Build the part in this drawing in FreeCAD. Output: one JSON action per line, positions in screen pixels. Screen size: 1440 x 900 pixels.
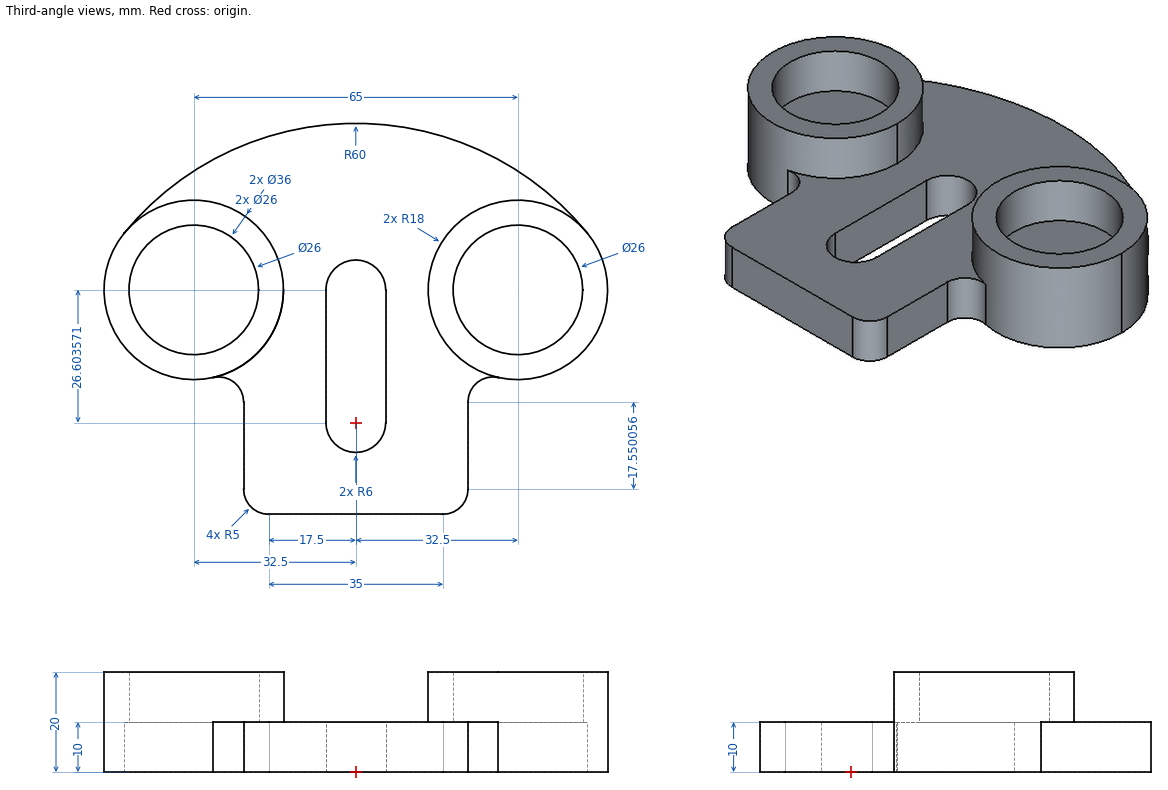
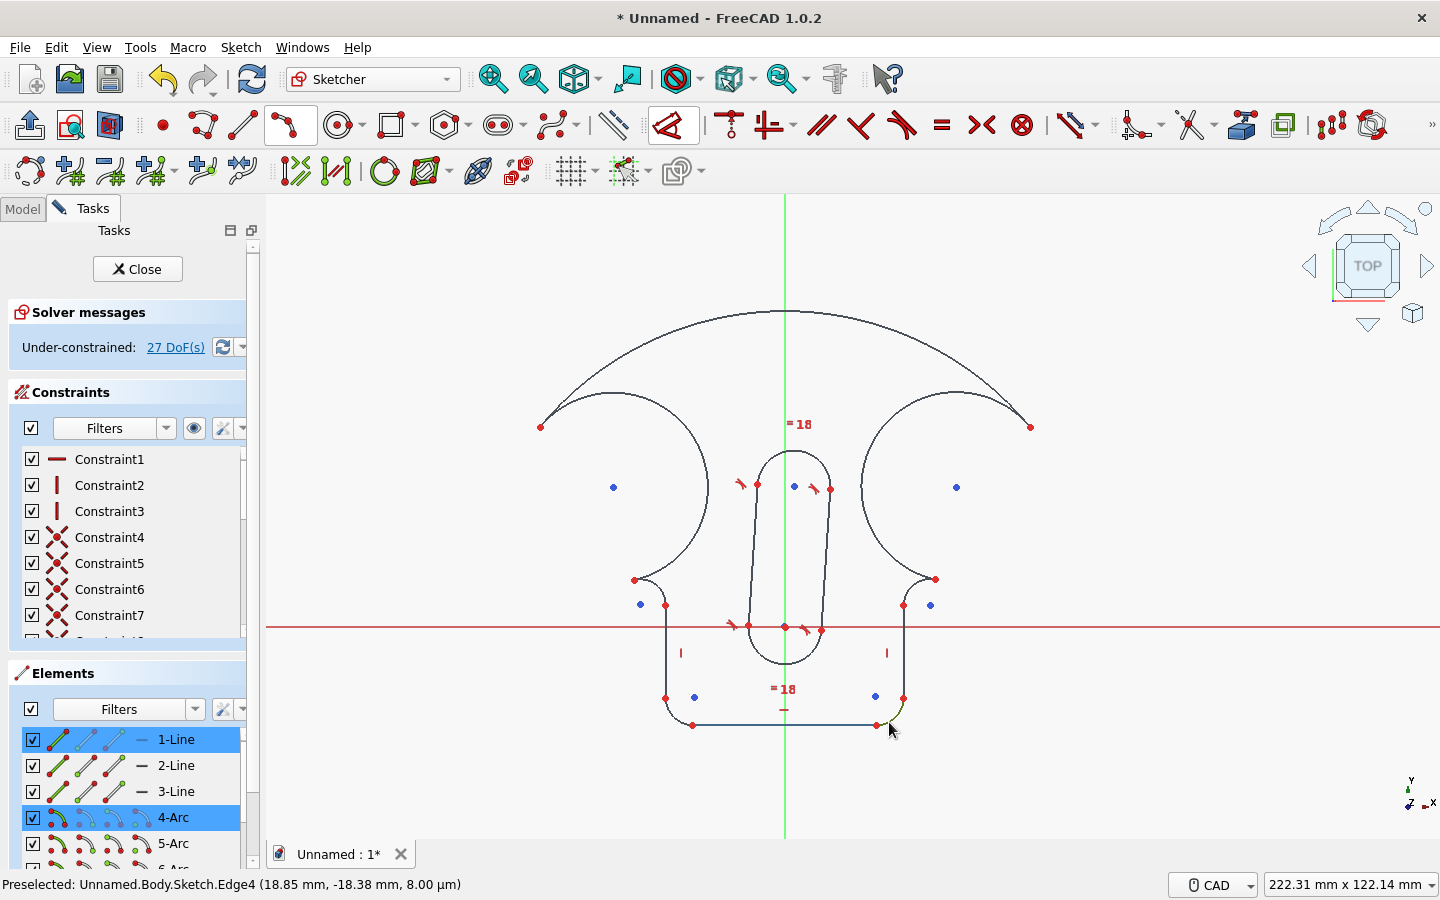
{"action": "left_click", "coordinate": [902, 126]}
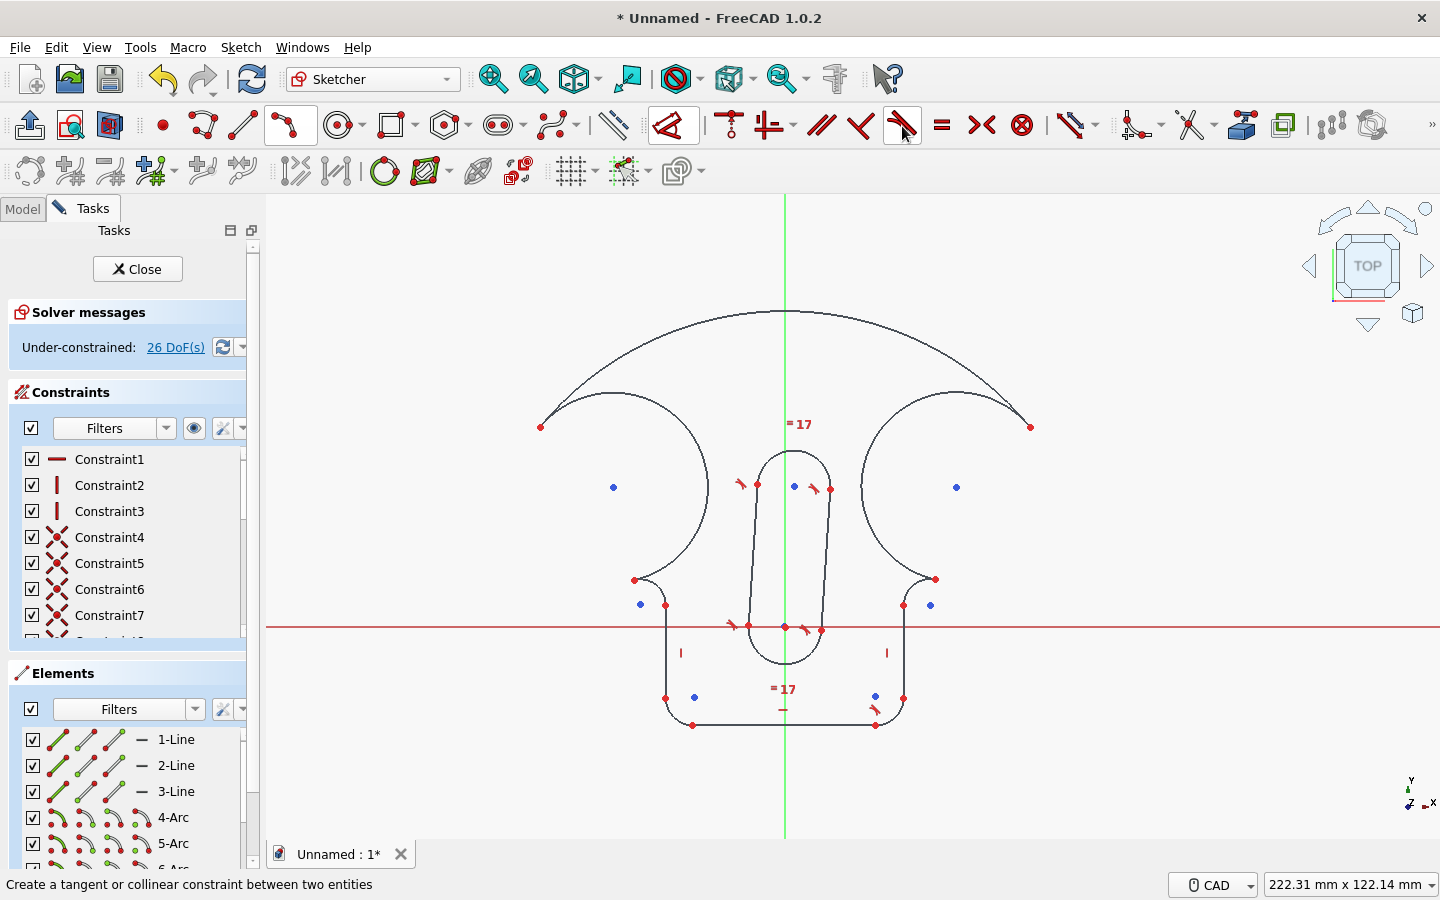
{"action": "left_click", "coordinate": [747, 725]}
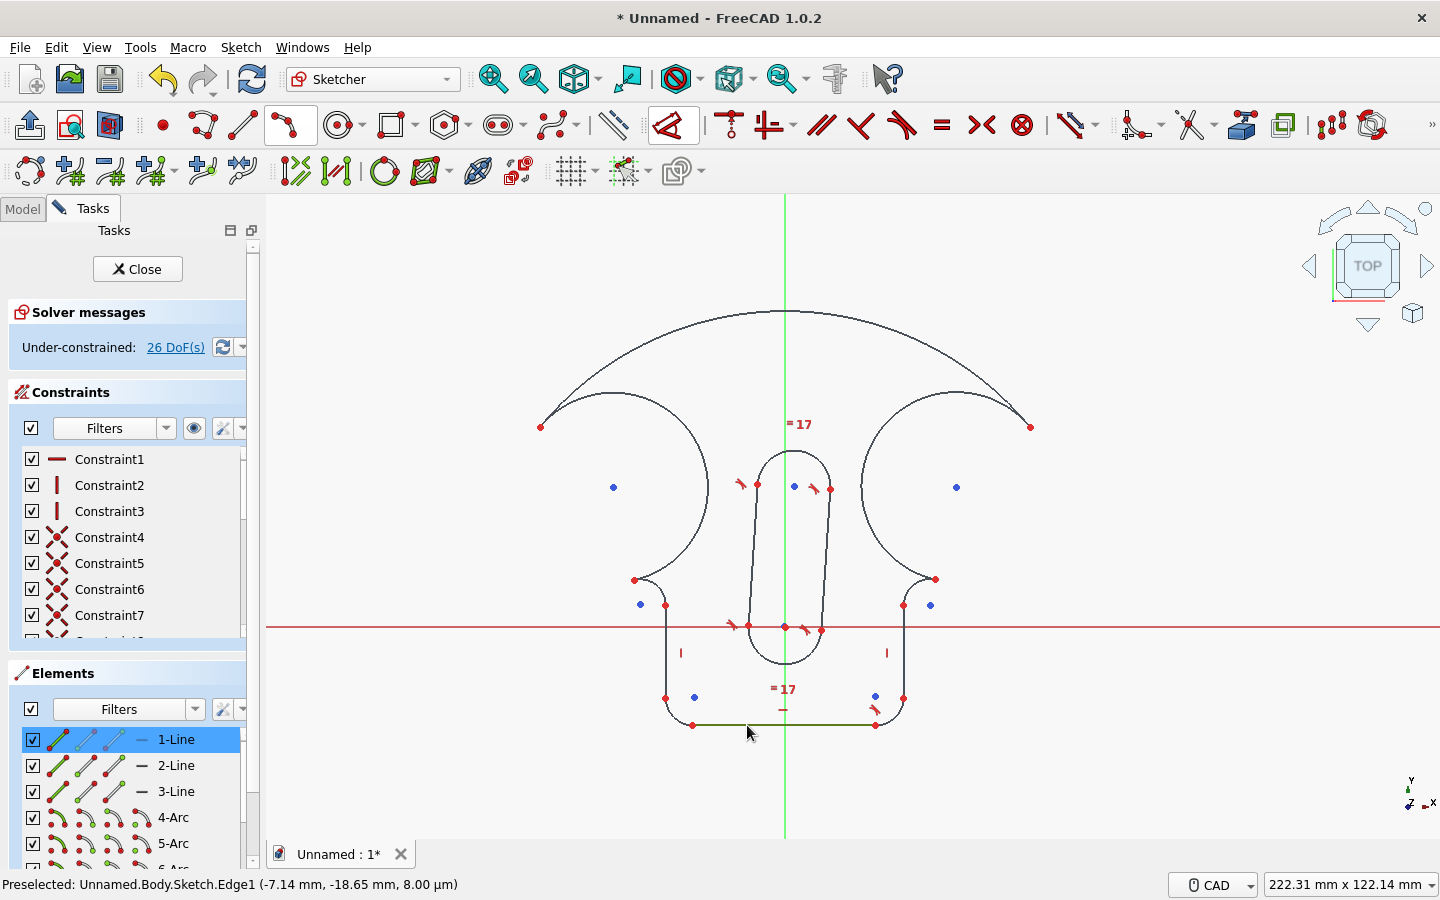
{"action": "left_click", "coordinate": [669, 710]}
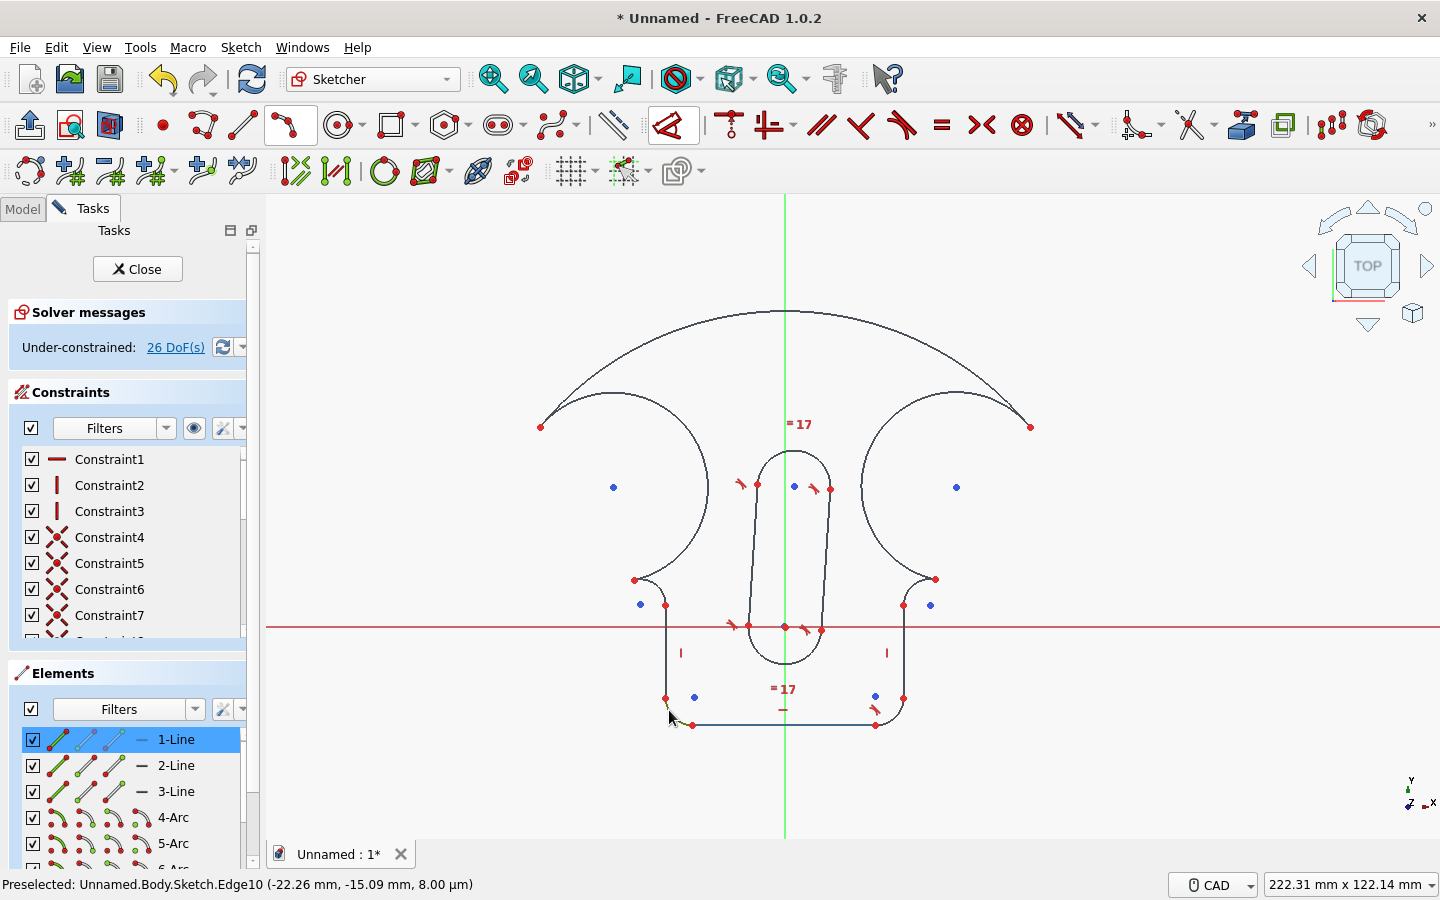
{"action": "key", "text": "t"}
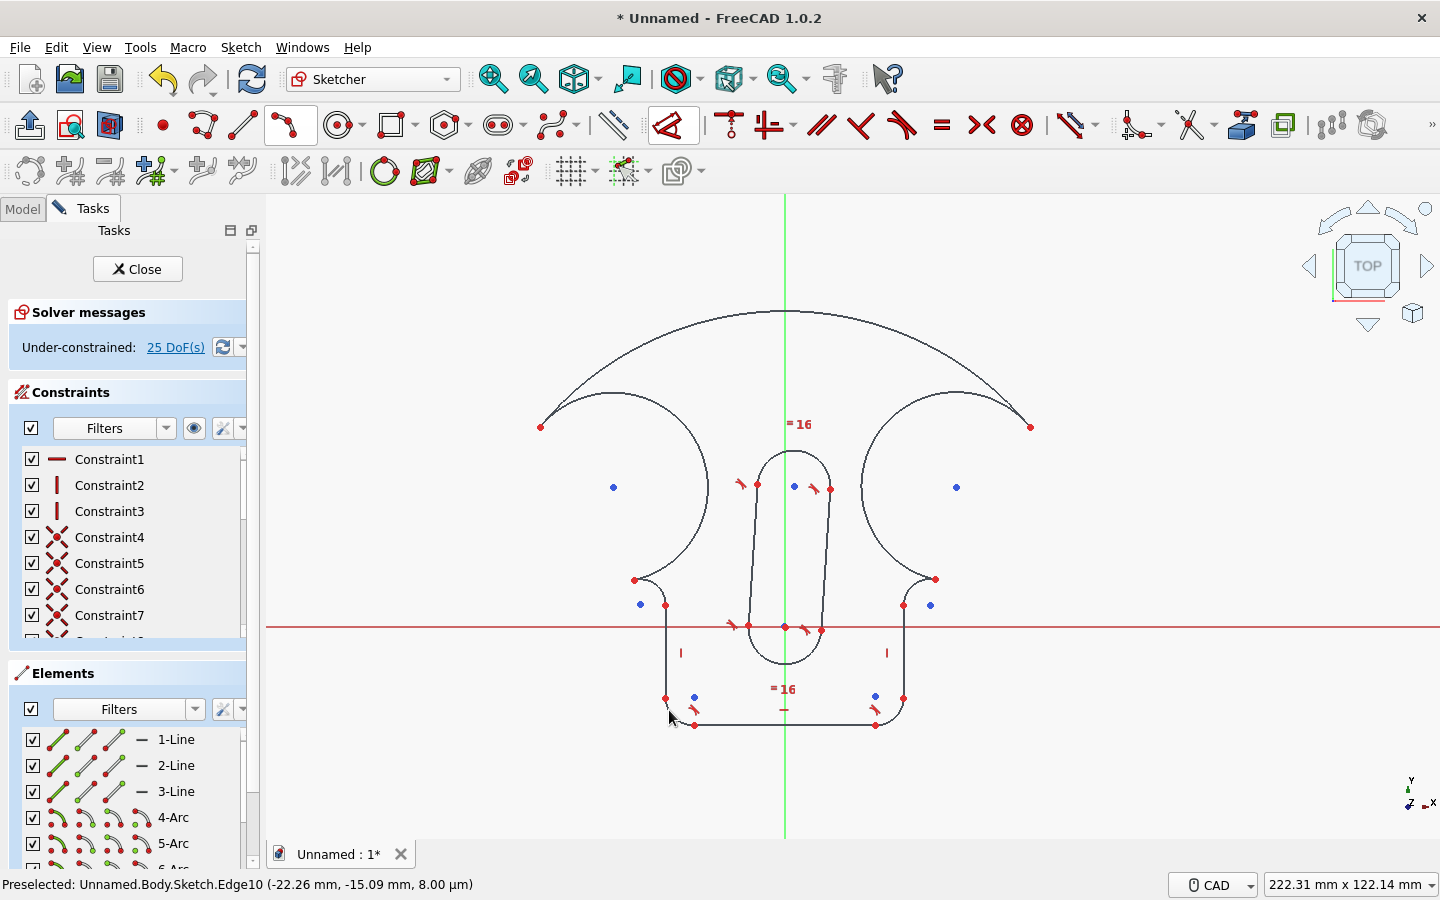
{"action": "left_click", "coordinate": [904, 671]}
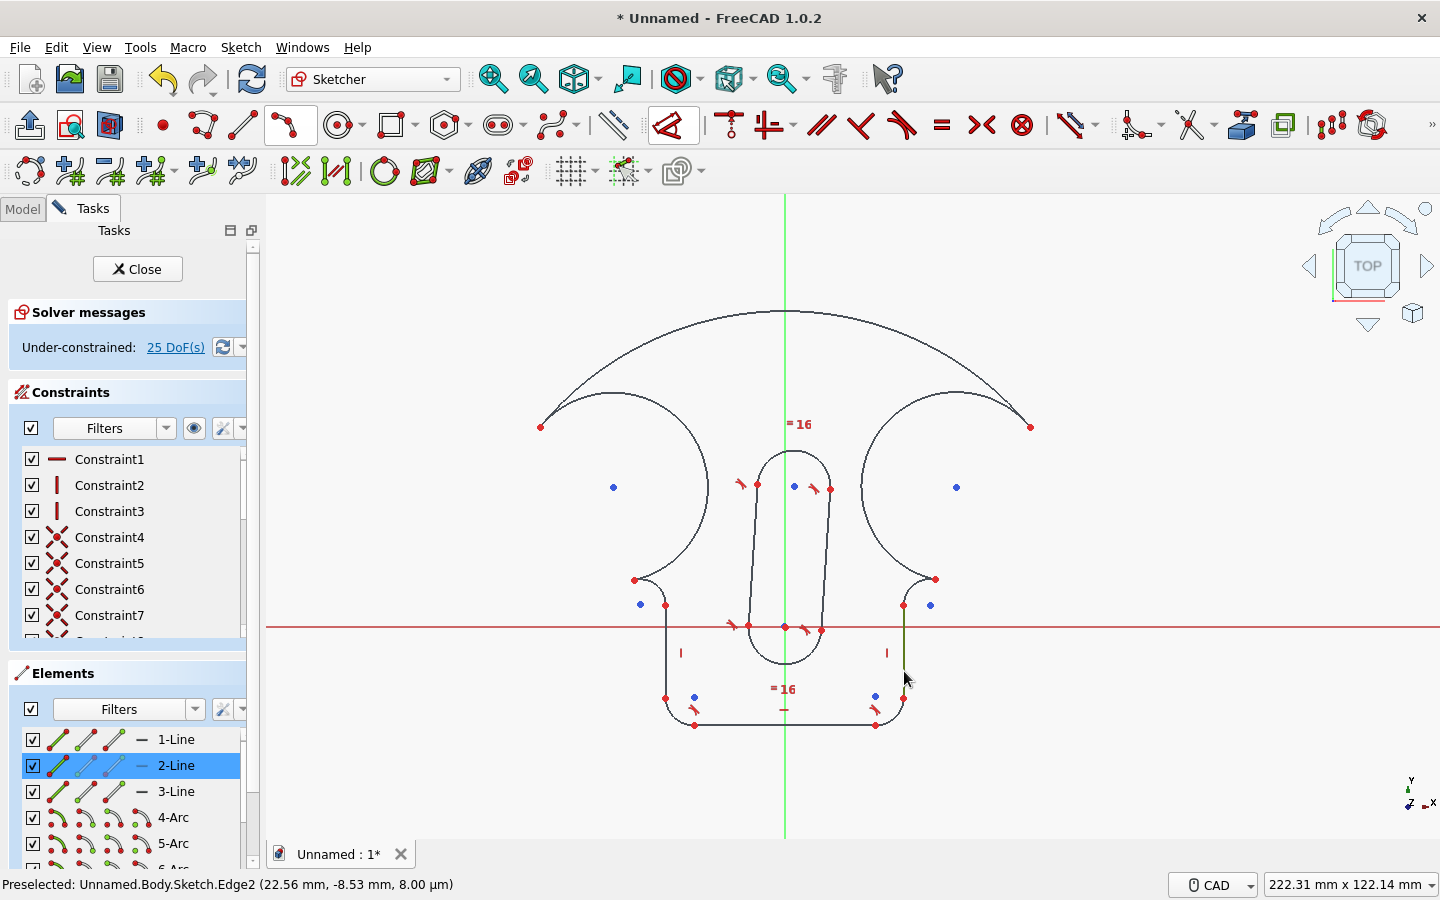
{"action": "left_click", "coordinate": [888, 723]}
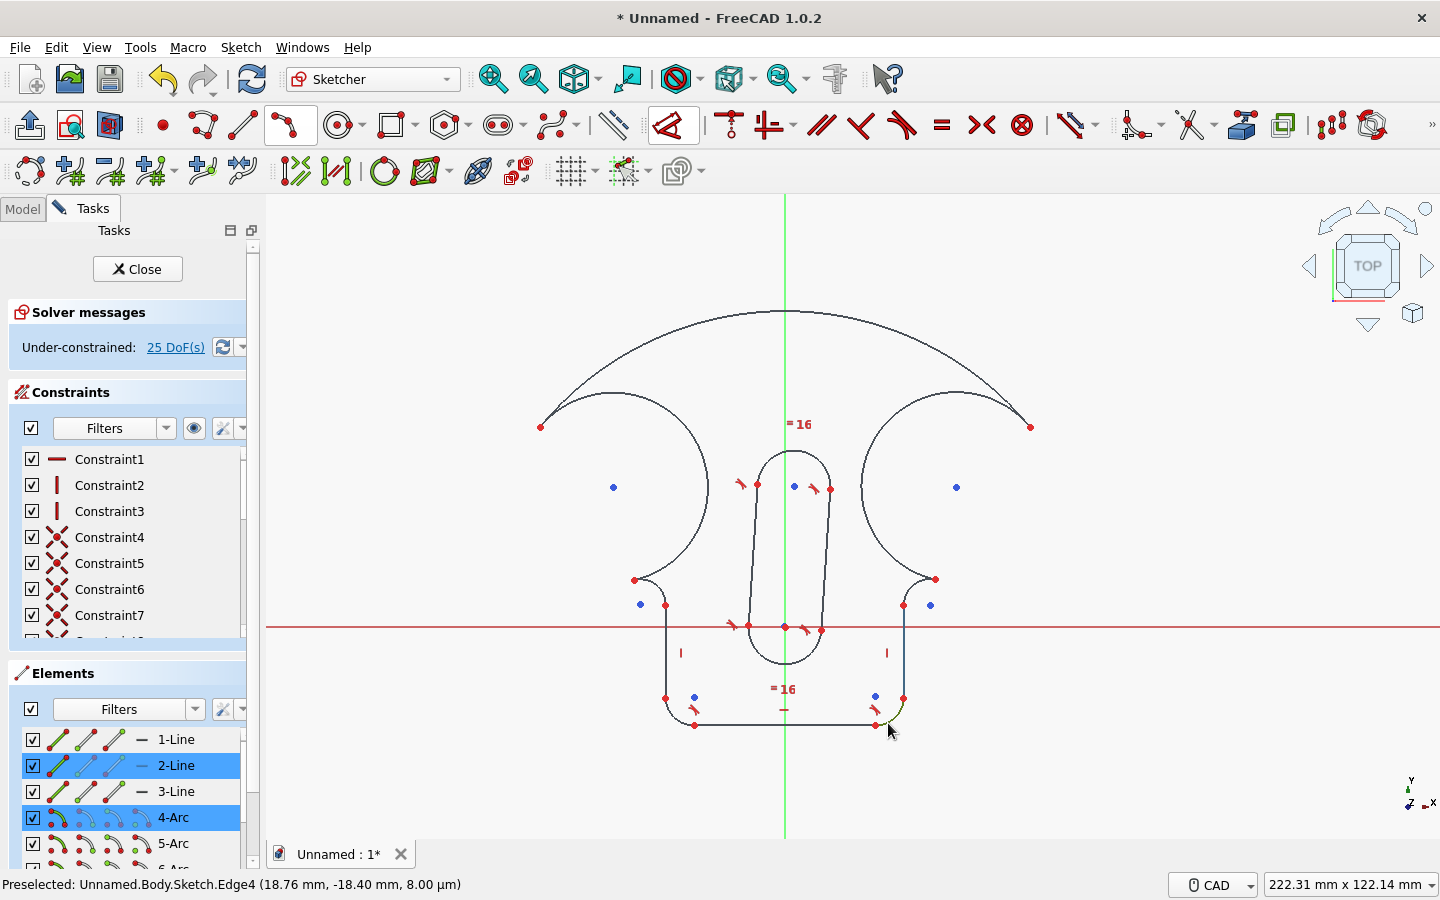
{"action": "left_click", "coordinate": [902, 126]}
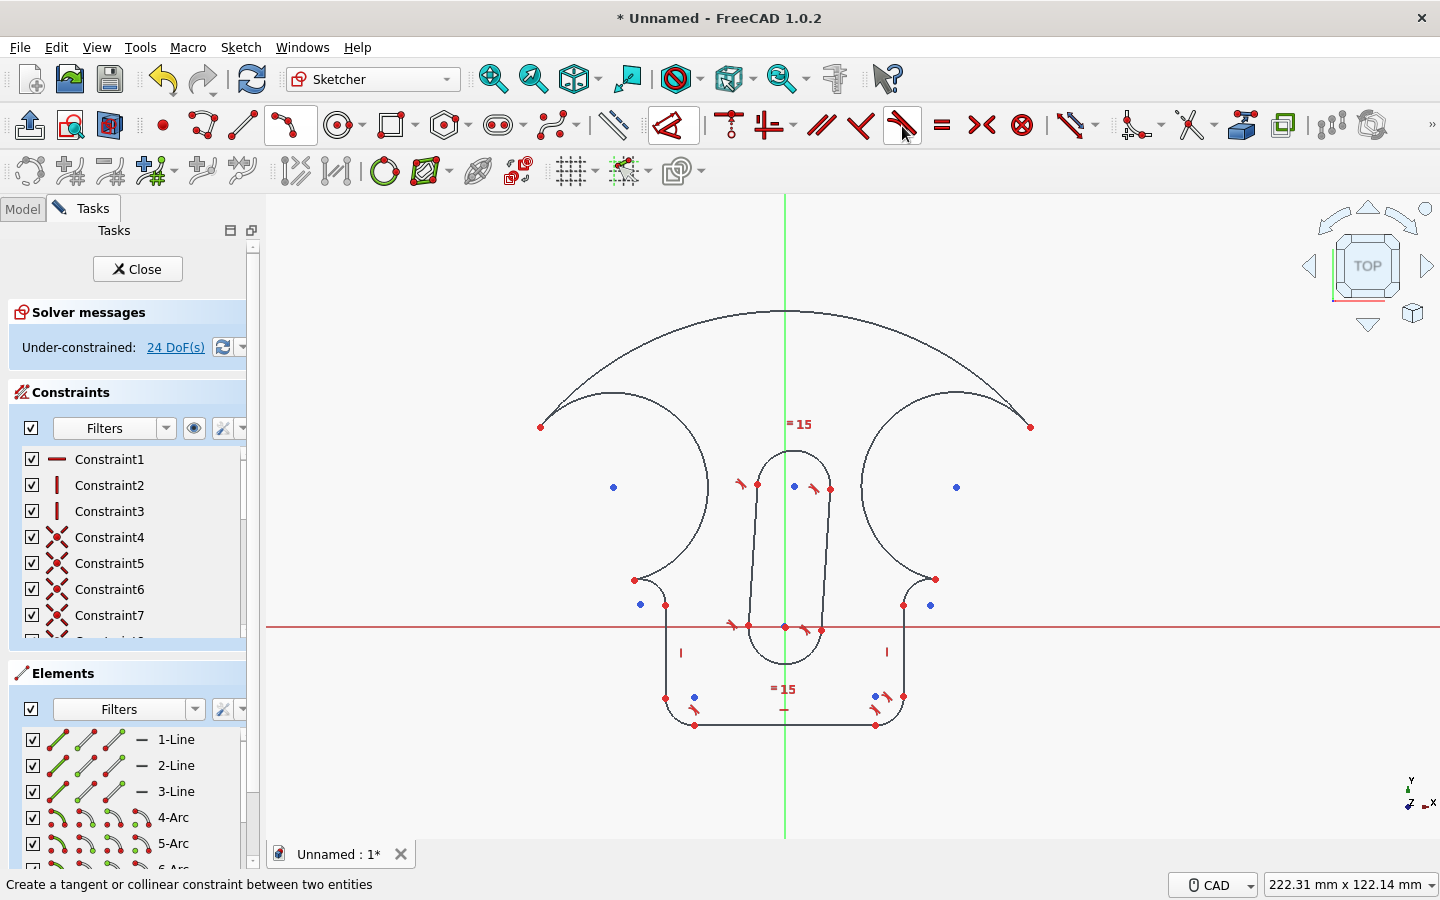
{"action": "left_click", "coordinate": [904, 670]}